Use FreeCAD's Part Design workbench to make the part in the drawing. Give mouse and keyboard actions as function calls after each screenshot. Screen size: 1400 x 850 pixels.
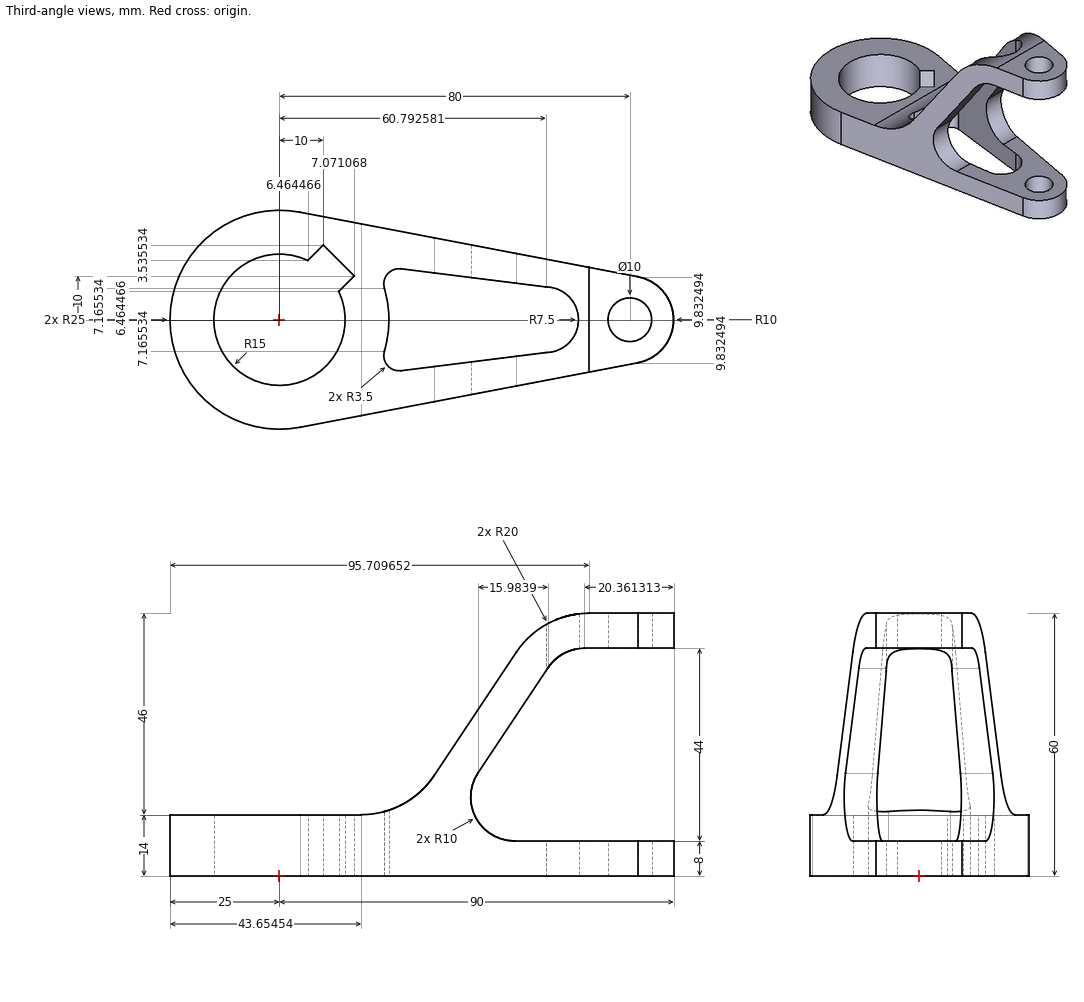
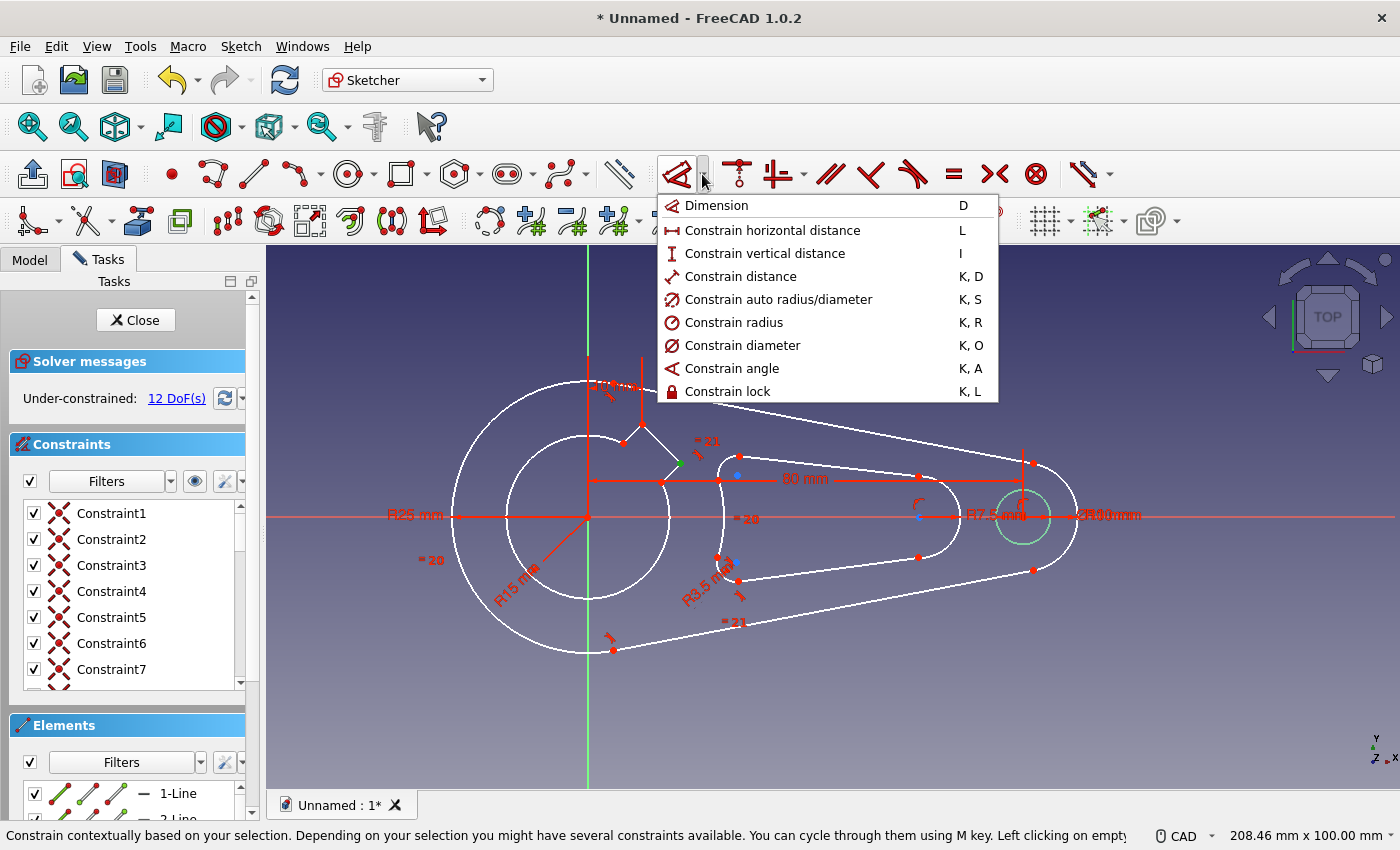
click(828, 254)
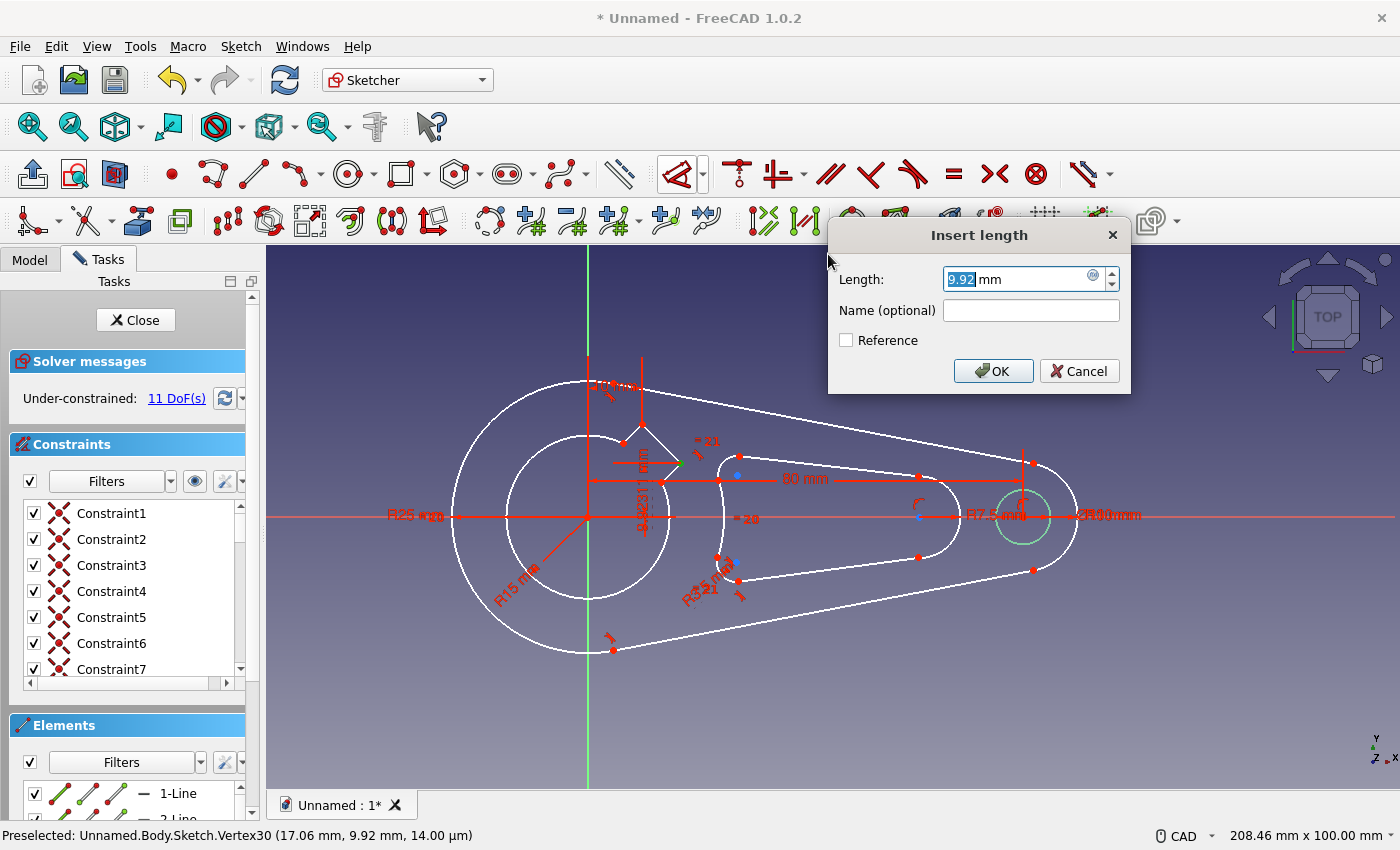
text(10)
key(Return)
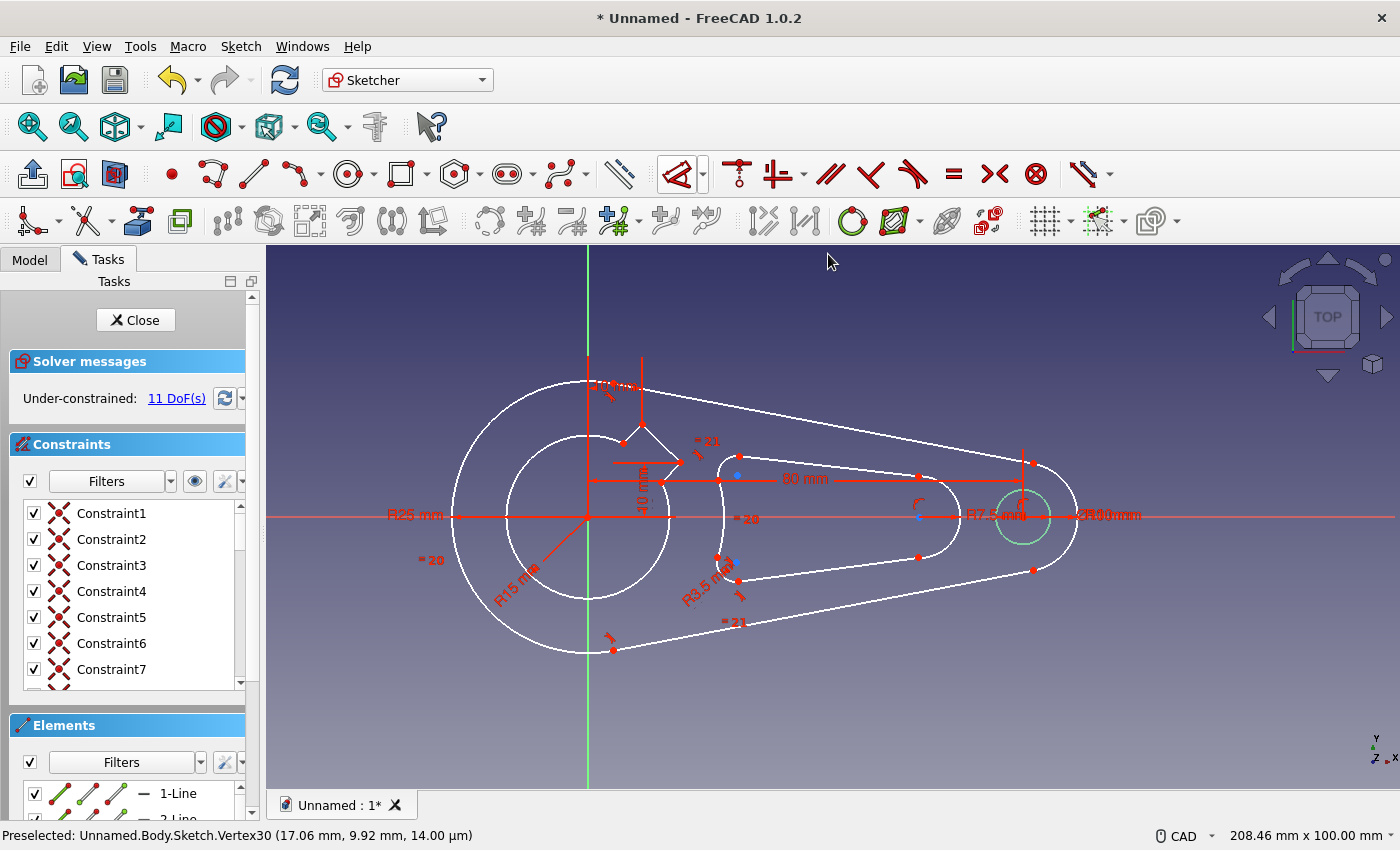
click(1033, 464)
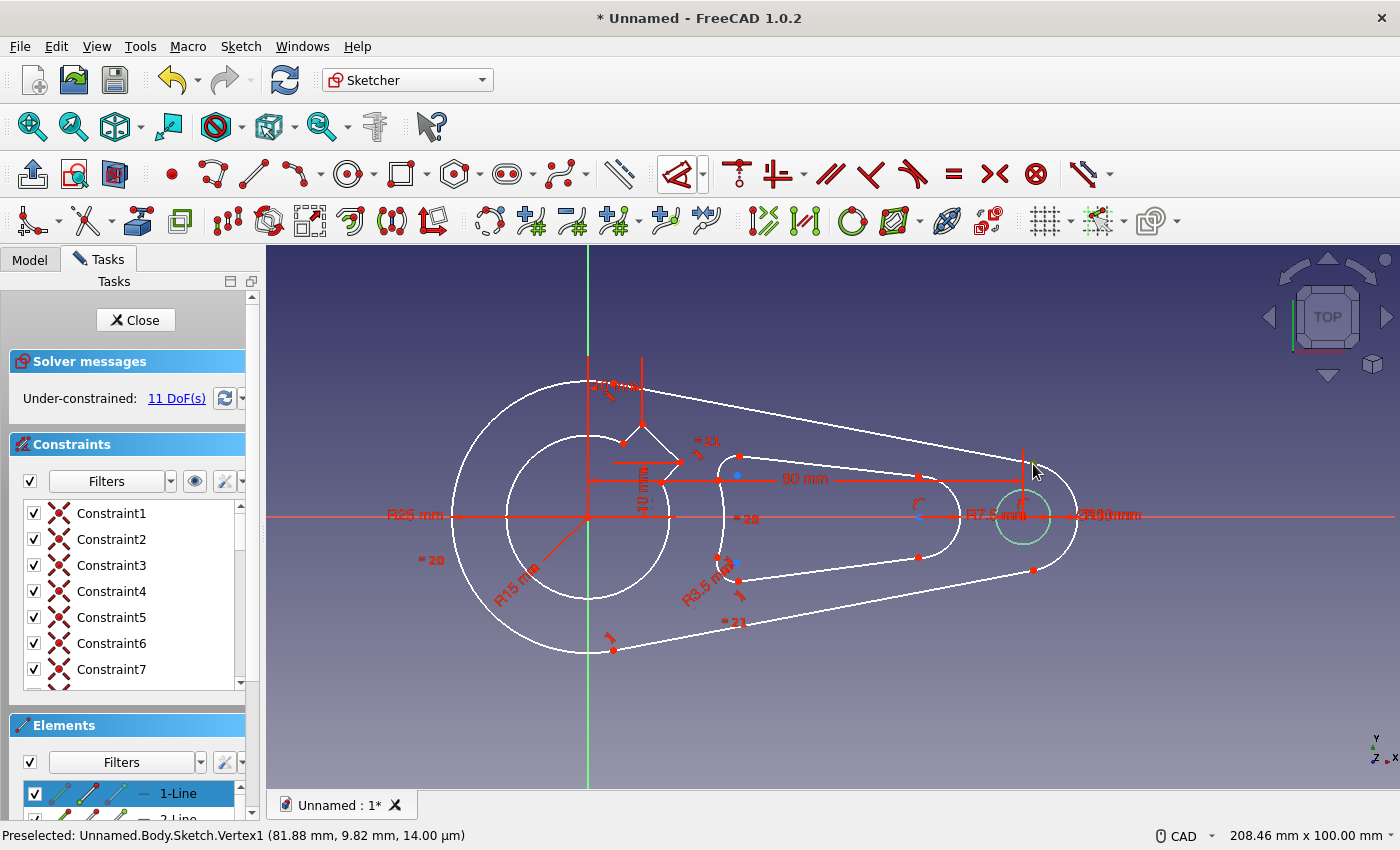
click(702, 174)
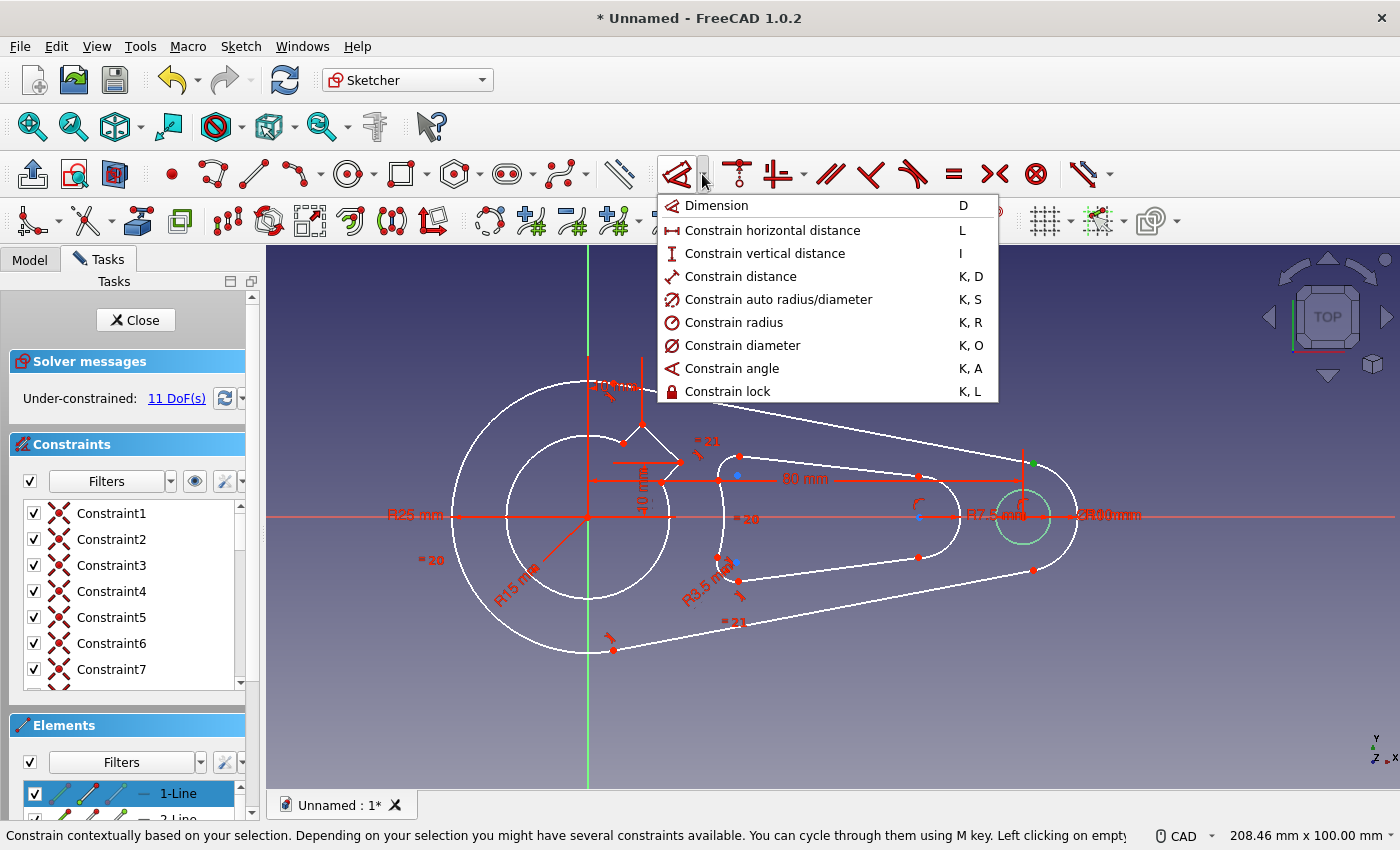
click(828, 254)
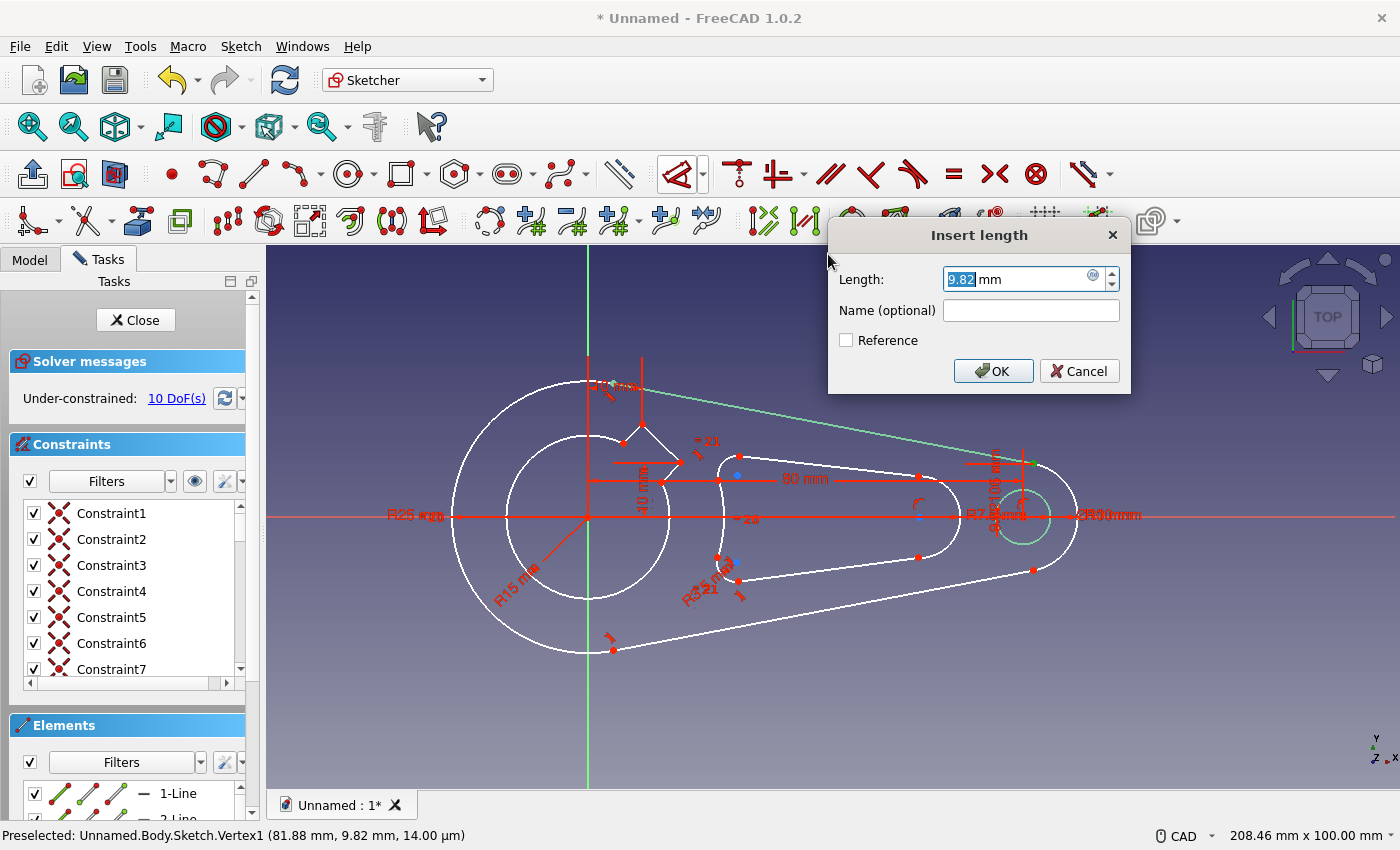
text(9.832494)
key(Return)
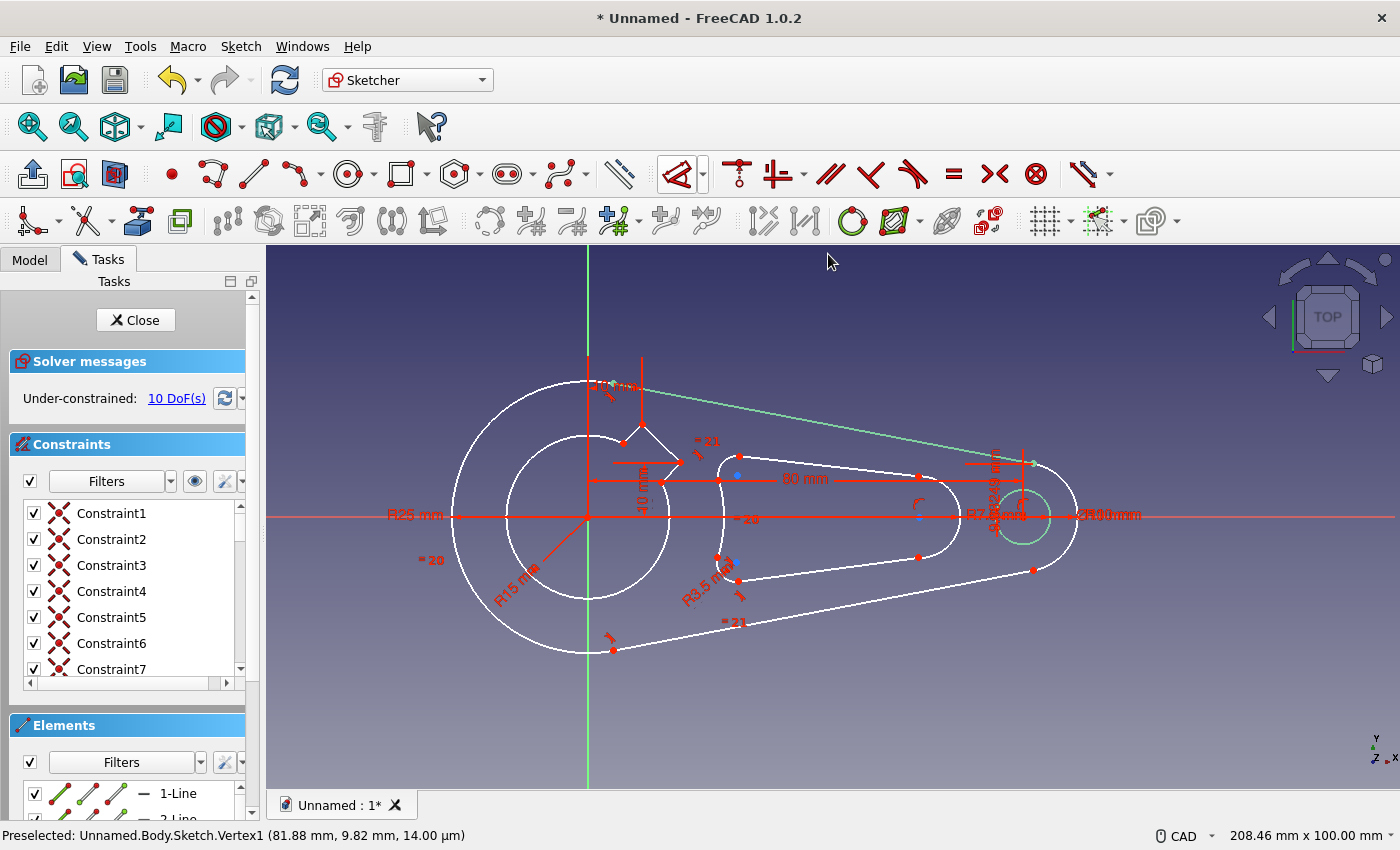
click(1033, 571)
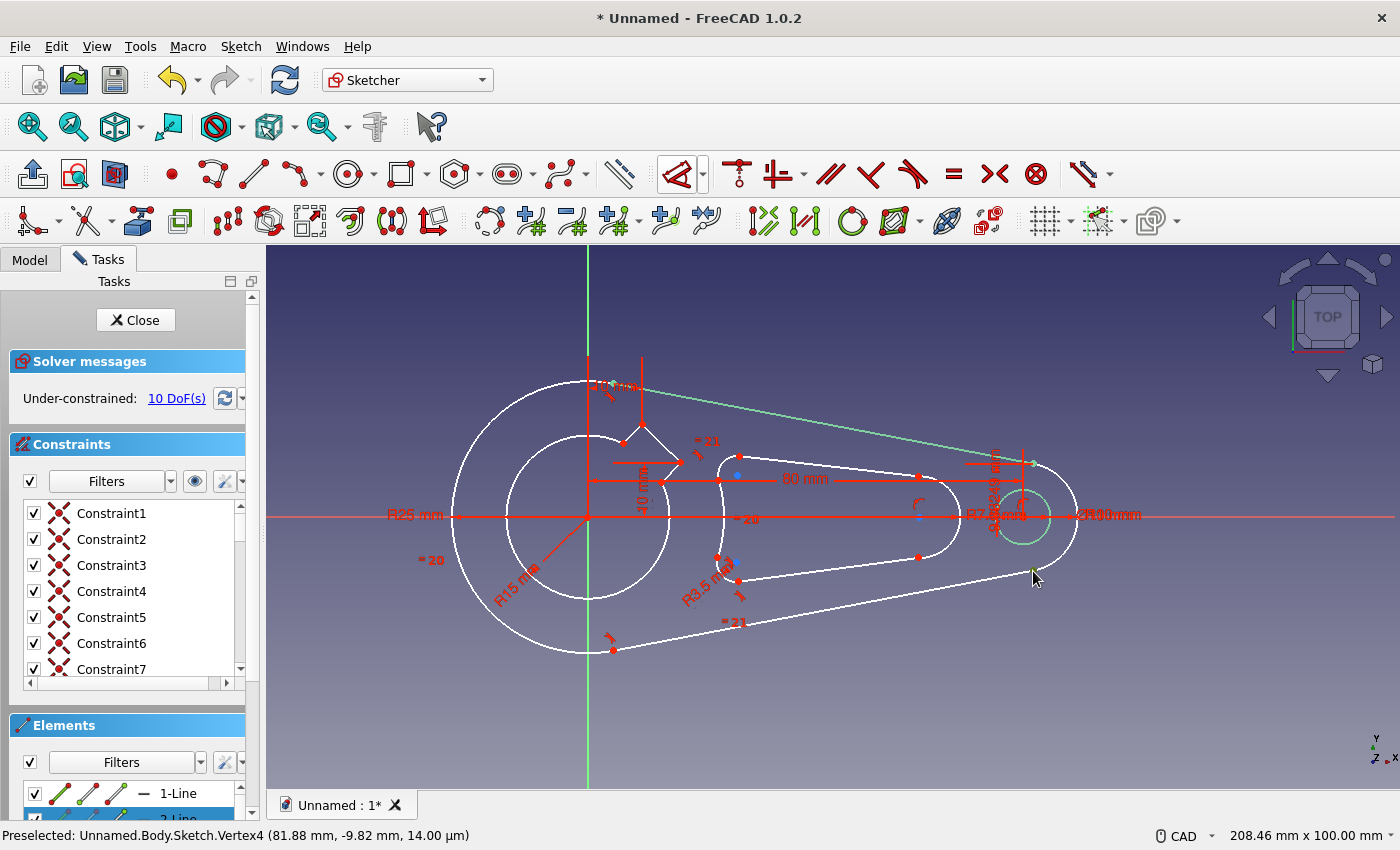
key(i)